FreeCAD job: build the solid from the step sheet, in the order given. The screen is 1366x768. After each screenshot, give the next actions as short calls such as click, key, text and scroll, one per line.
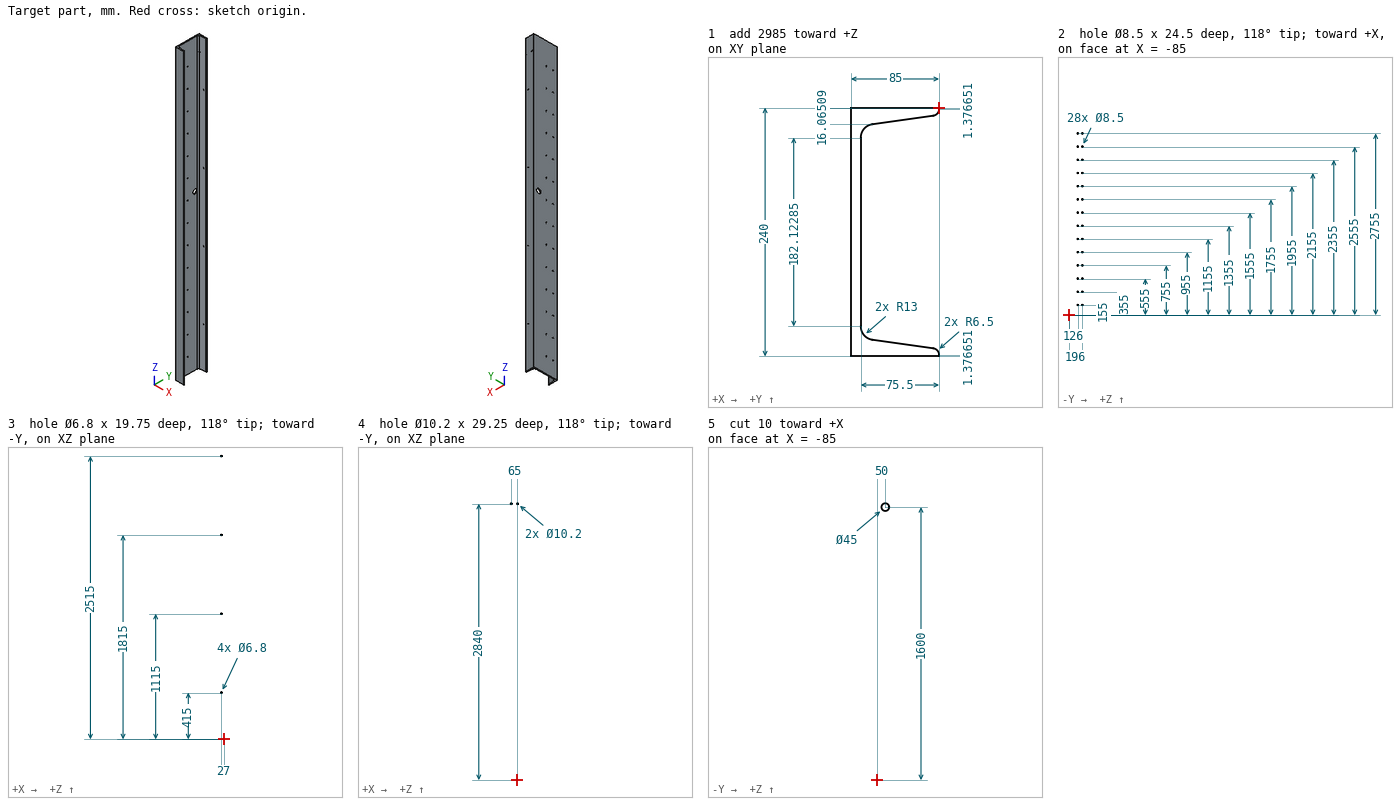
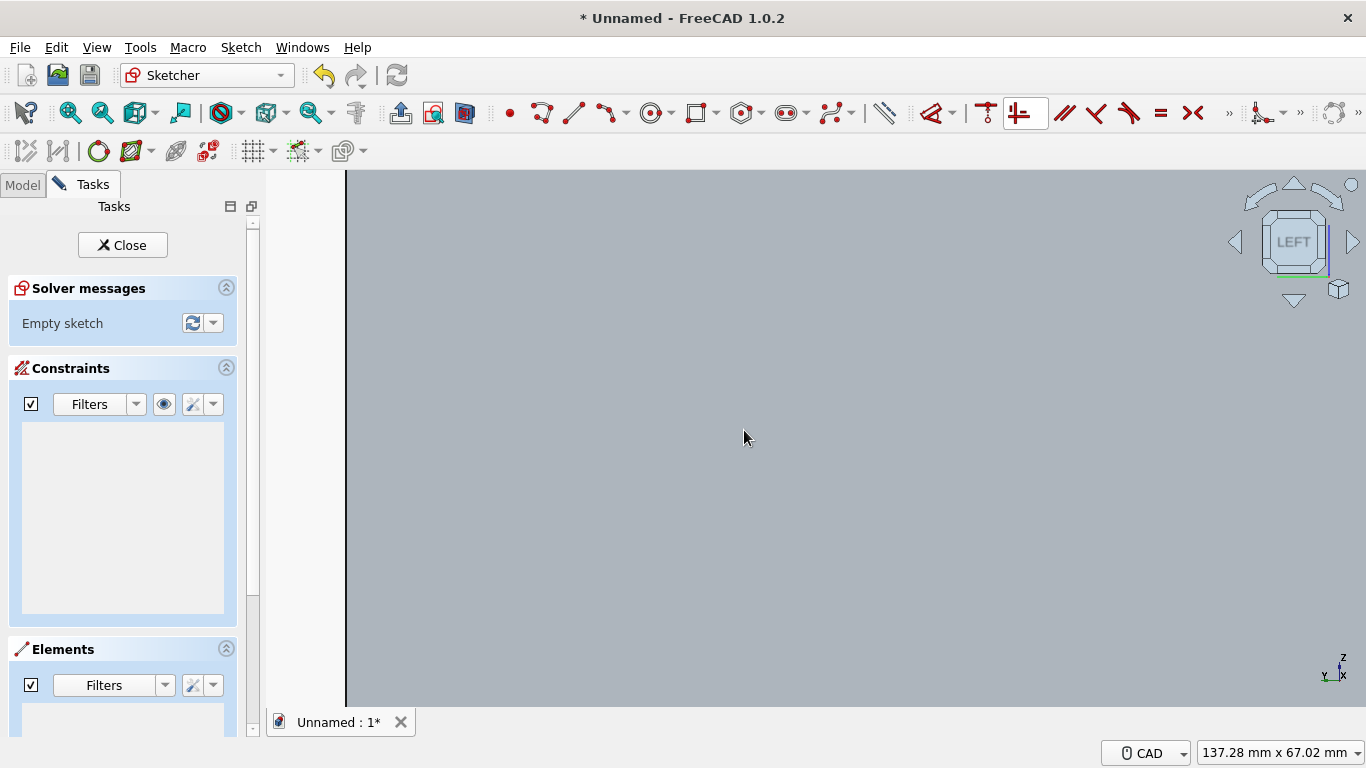
click(652, 114)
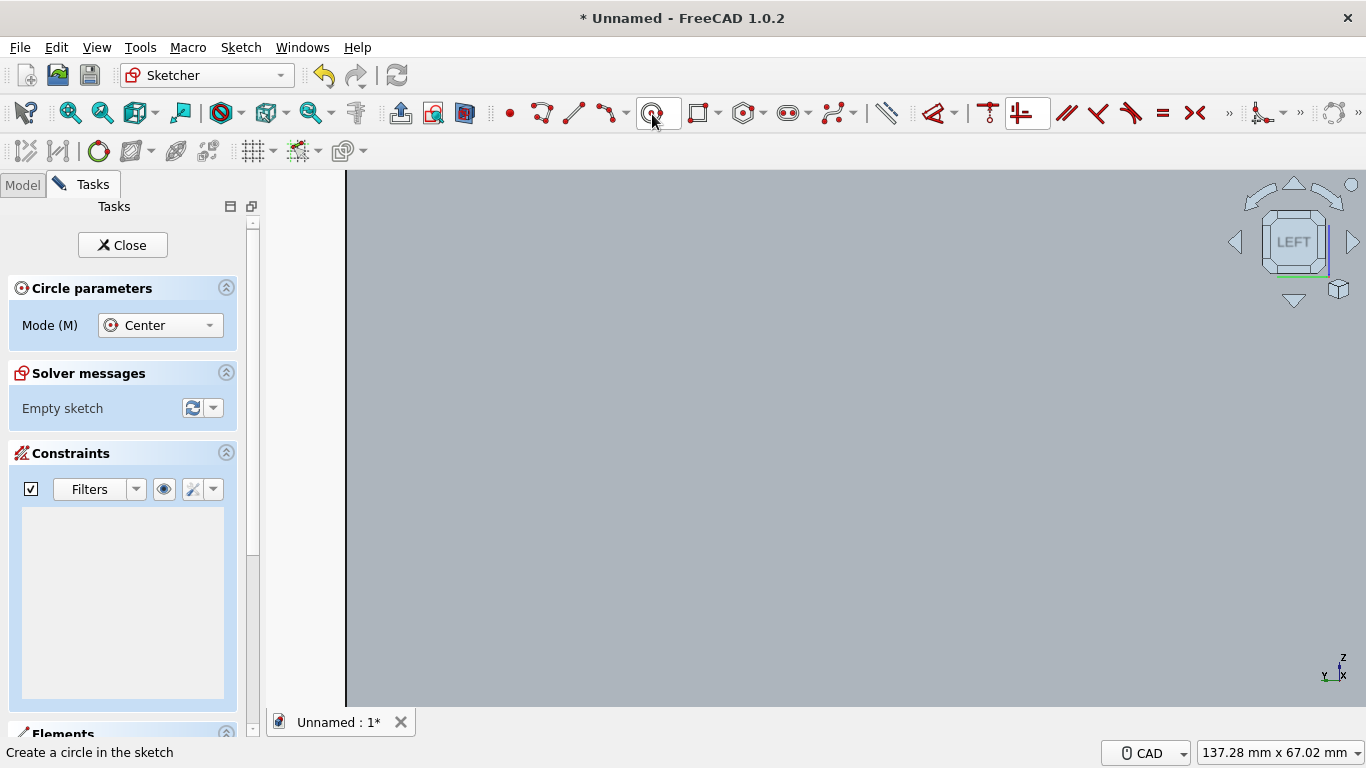
click(747, 438)
move(874, 311)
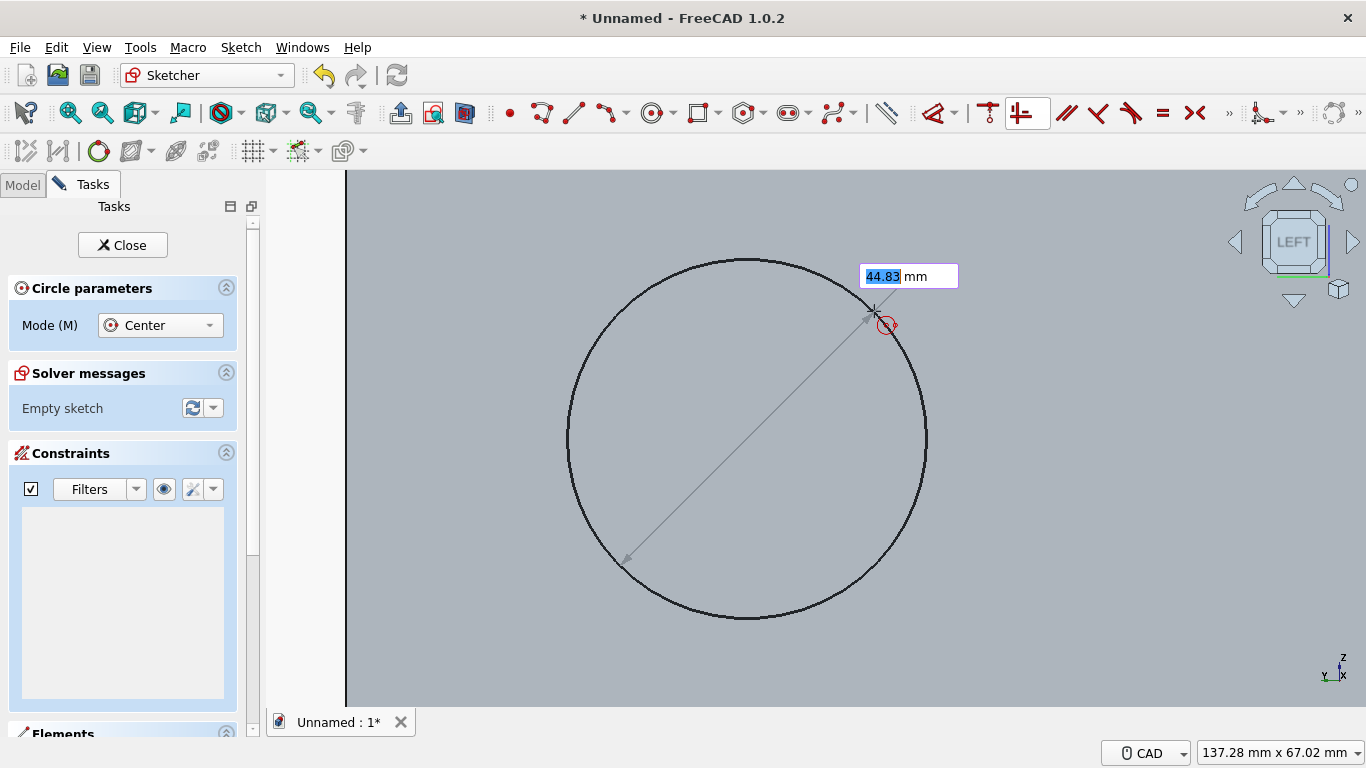
text(45)
key(Return)
key(Escape)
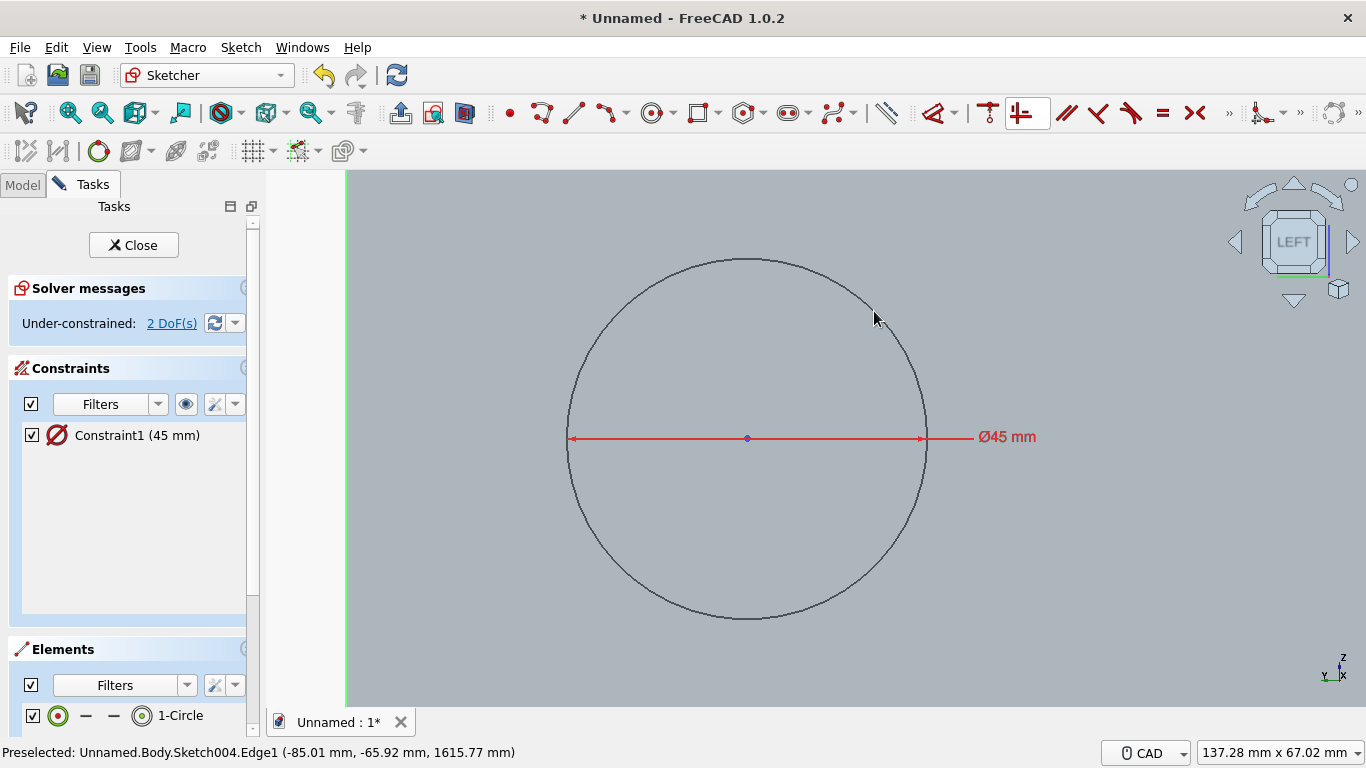
click(934, 114)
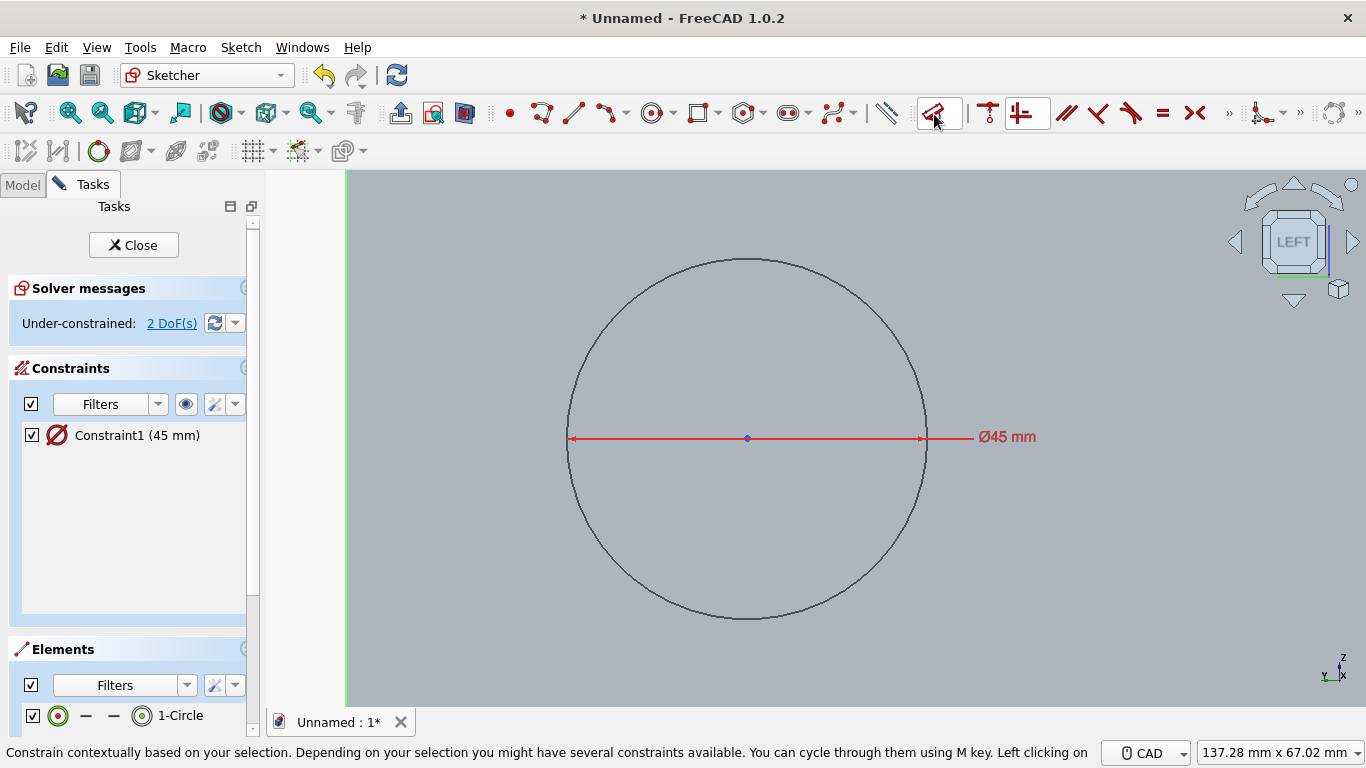
click(747, 439)
click(547, 405)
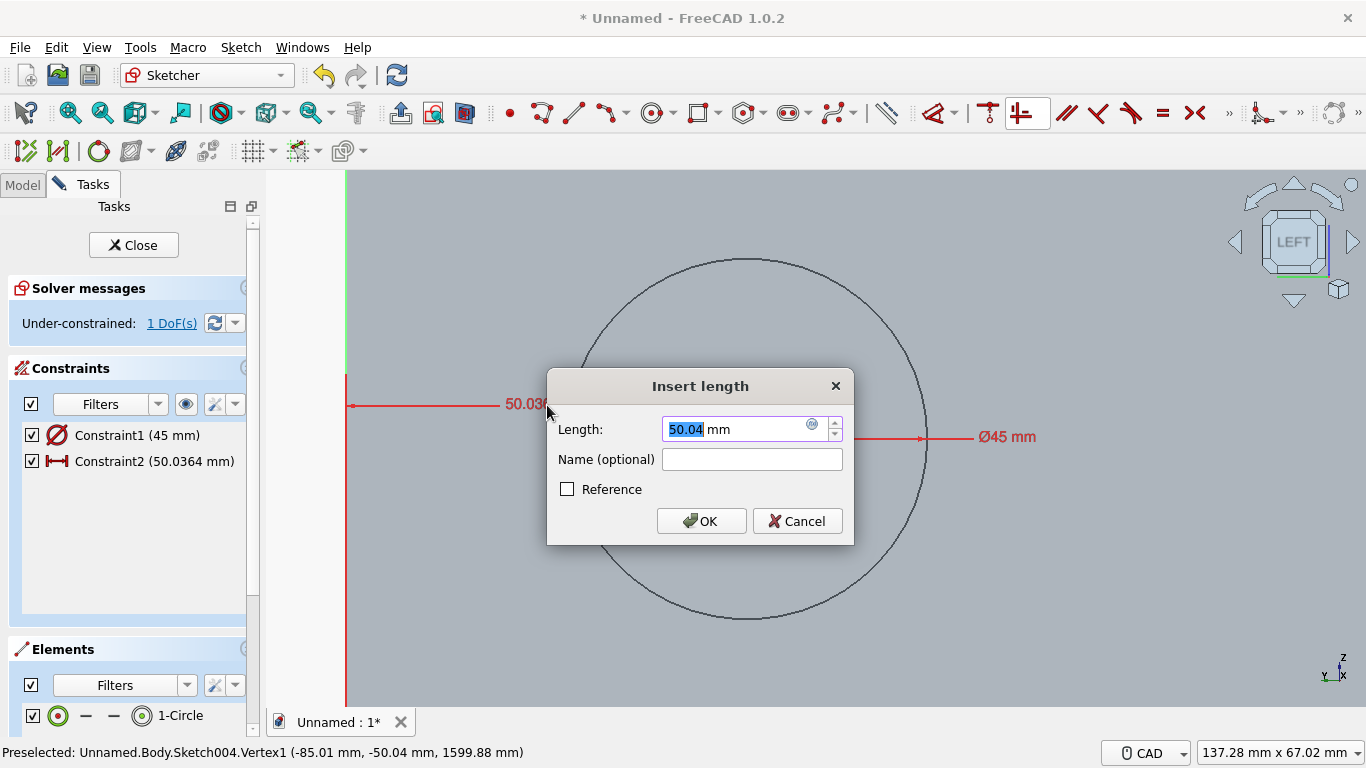
text(50)
key(Return)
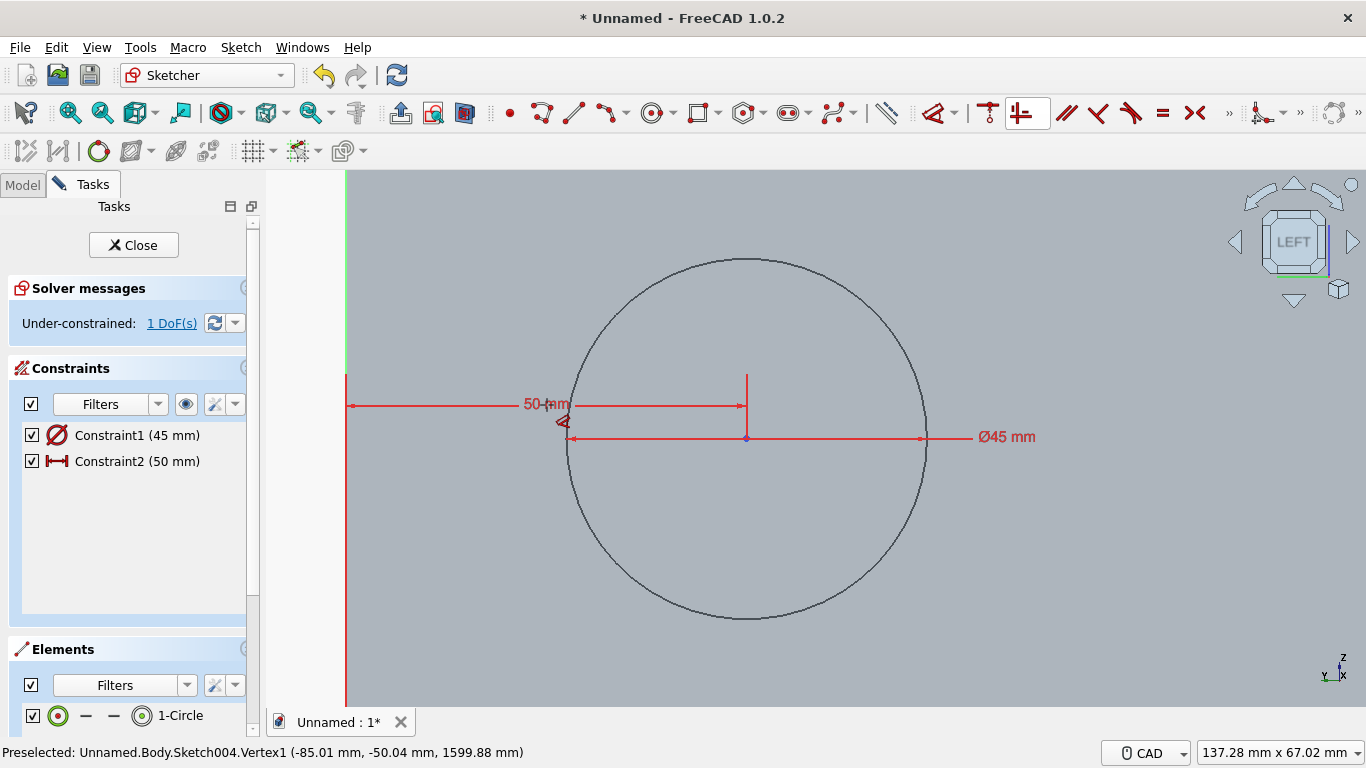
click(747, 439)
click(312, 559)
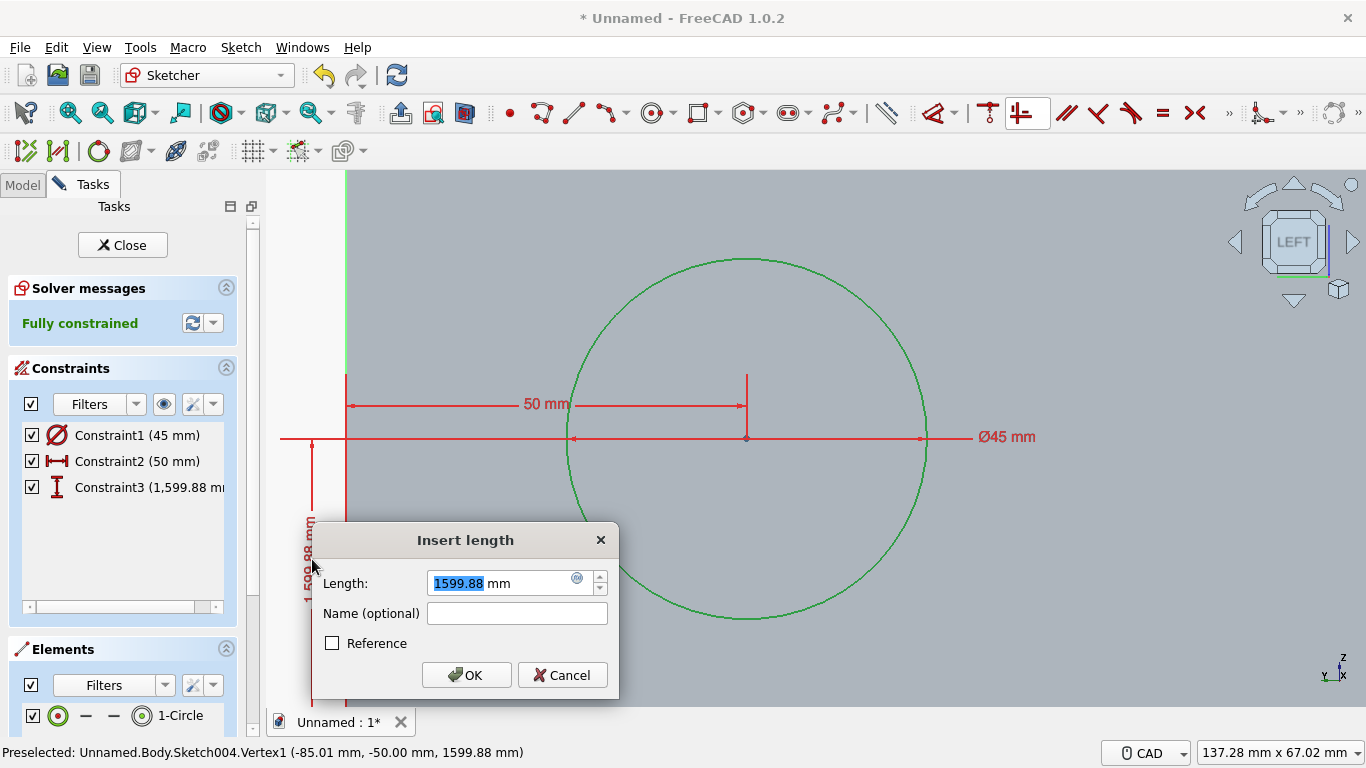
text(1600)
key(Return)
key(Escape)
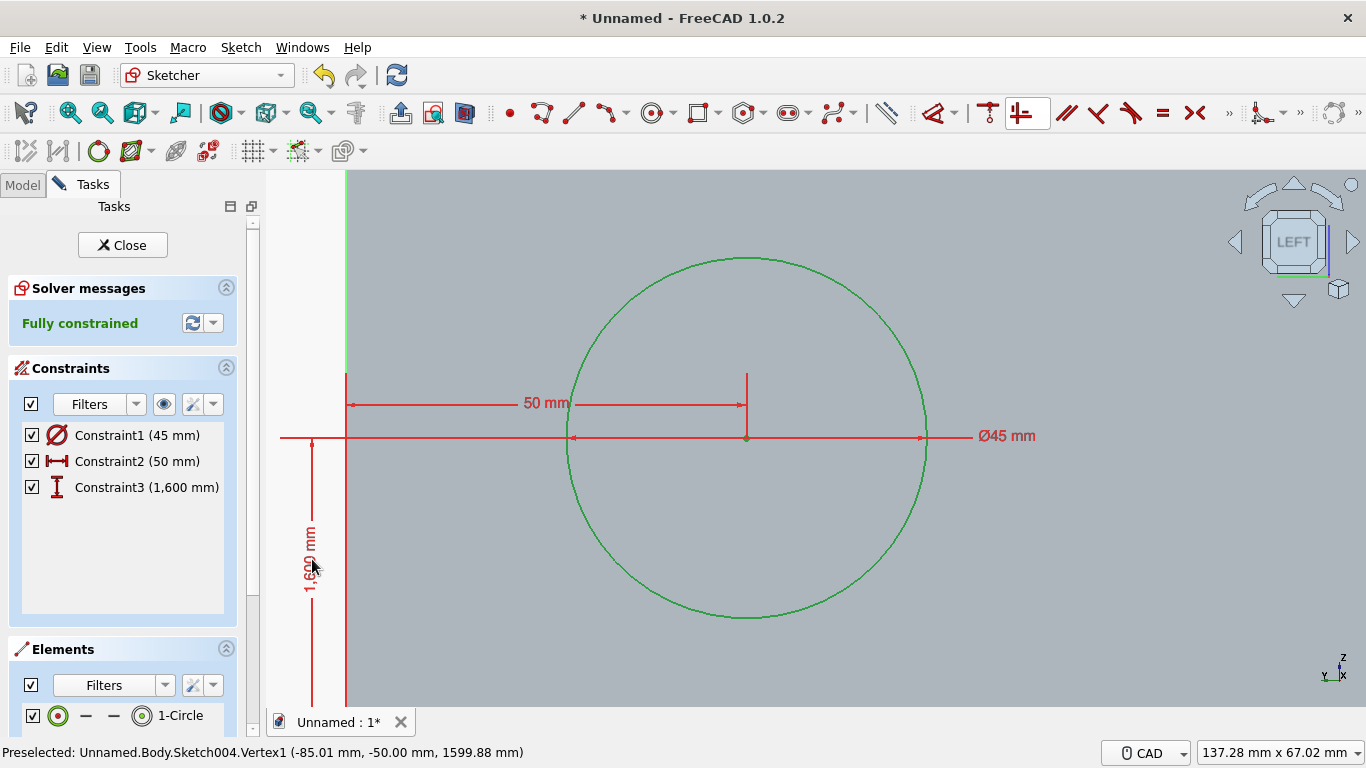
click(123, 245)